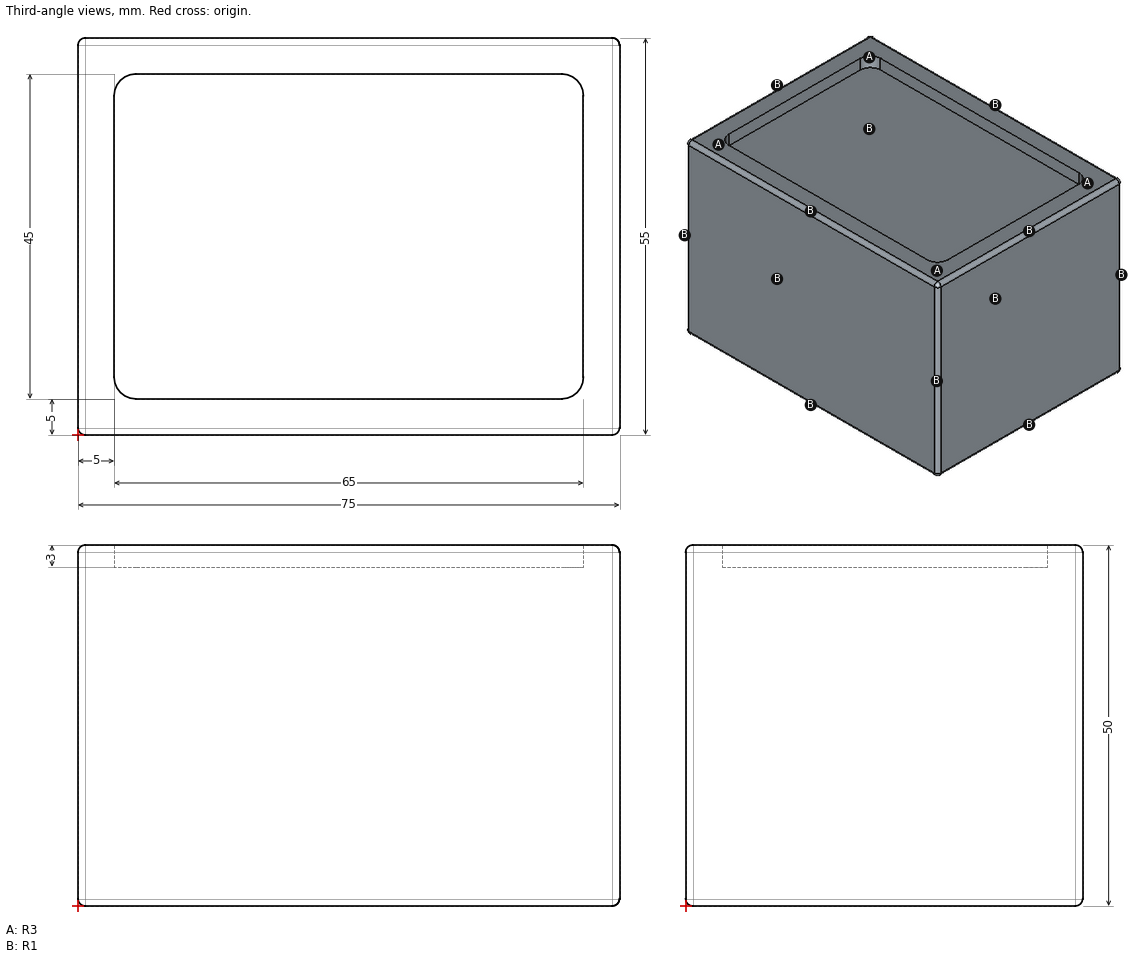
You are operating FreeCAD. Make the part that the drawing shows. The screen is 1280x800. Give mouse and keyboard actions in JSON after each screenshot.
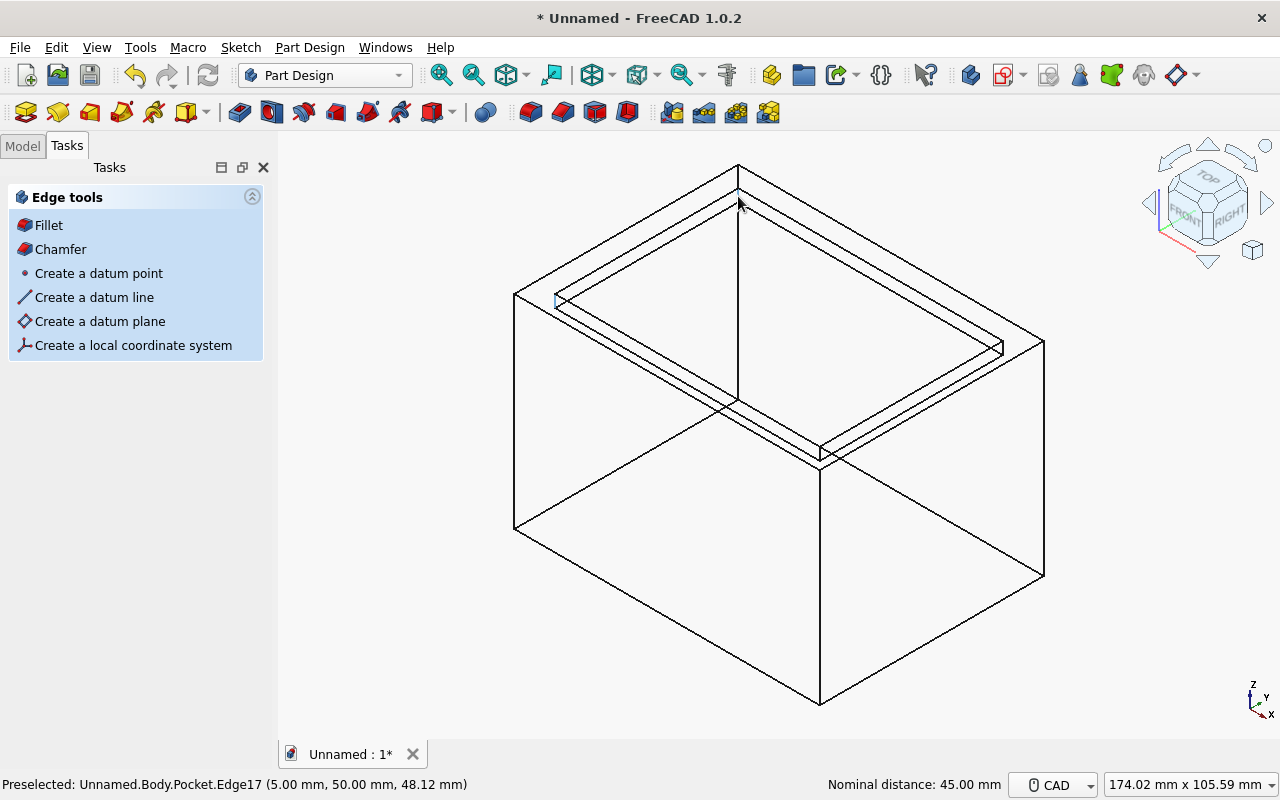
{"action": "left_click", "coordinate": [1003, 348], "text": "ctrl"}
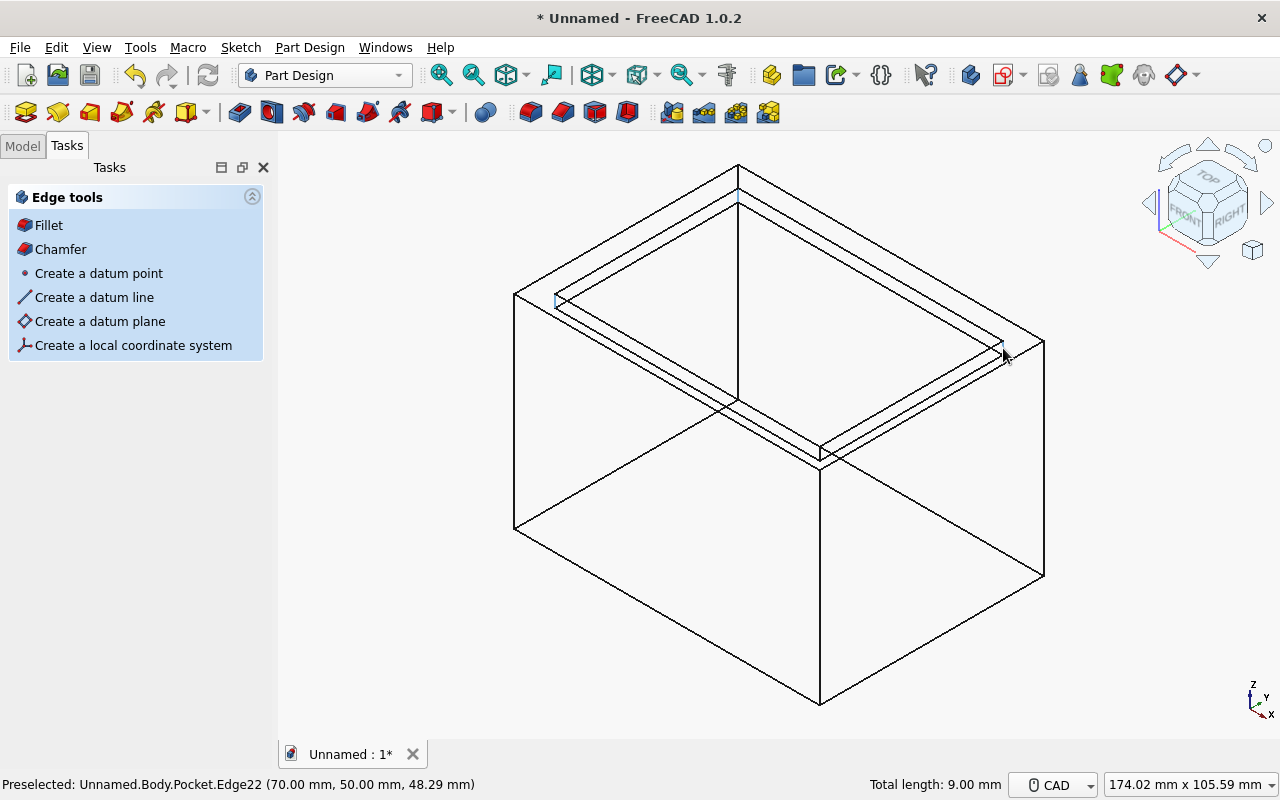
{"action": "left_click", "coordinate": [820, 453], "text": "ctrl"}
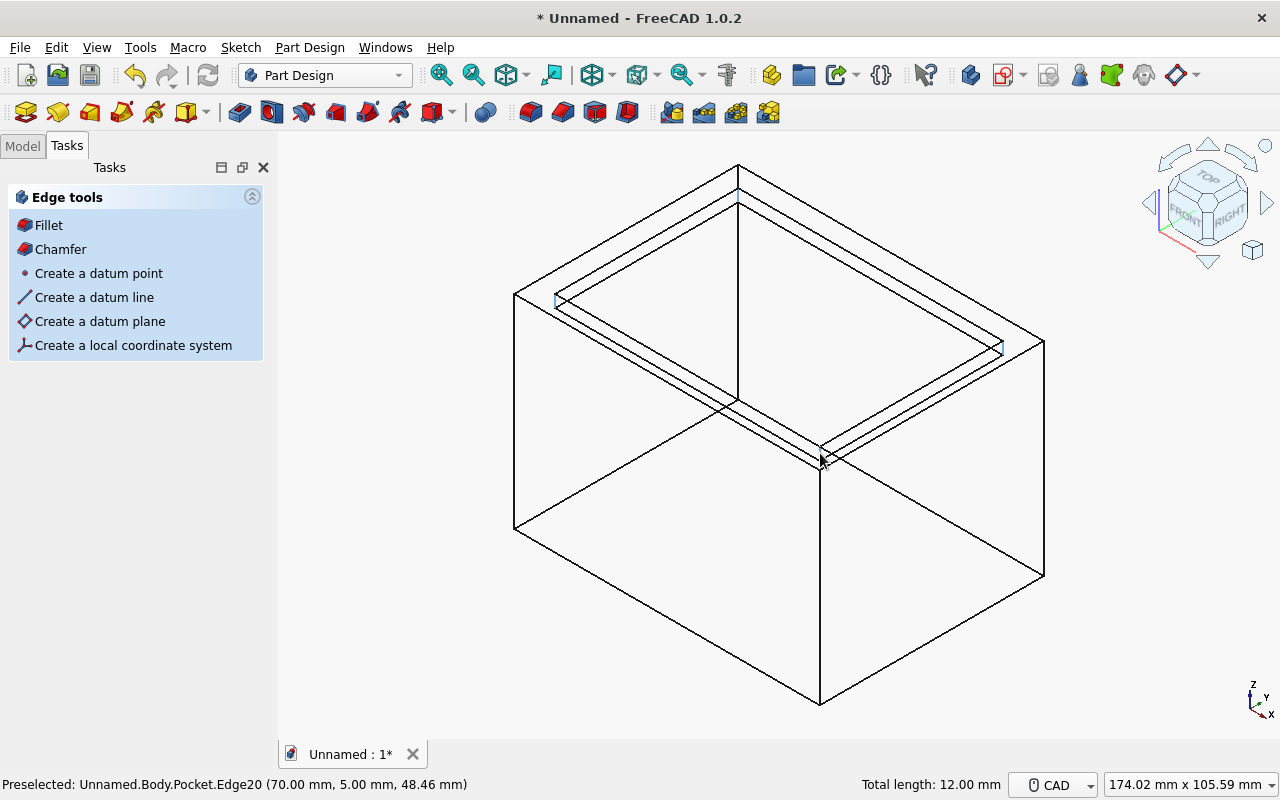
{"action": "key", "text": "v 1"}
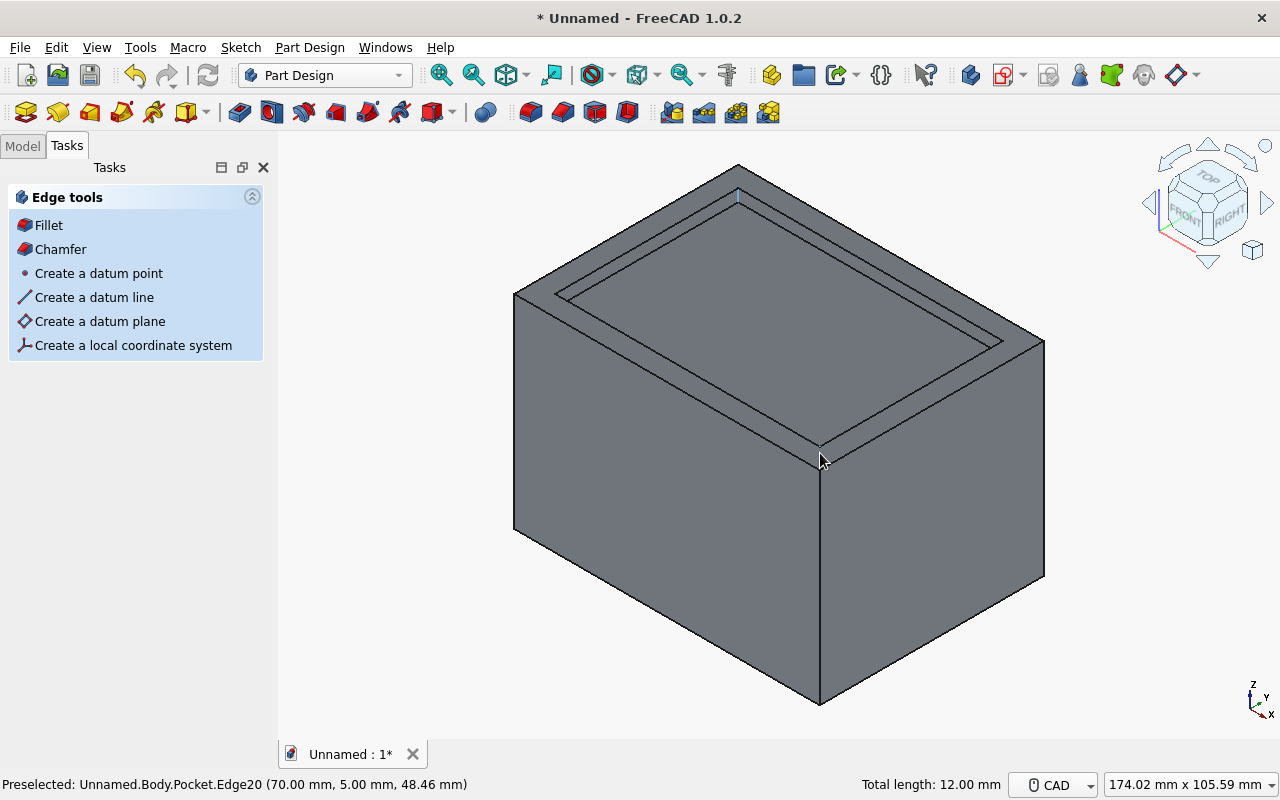
{"action": "left_click", "coordinate": [532, 112]}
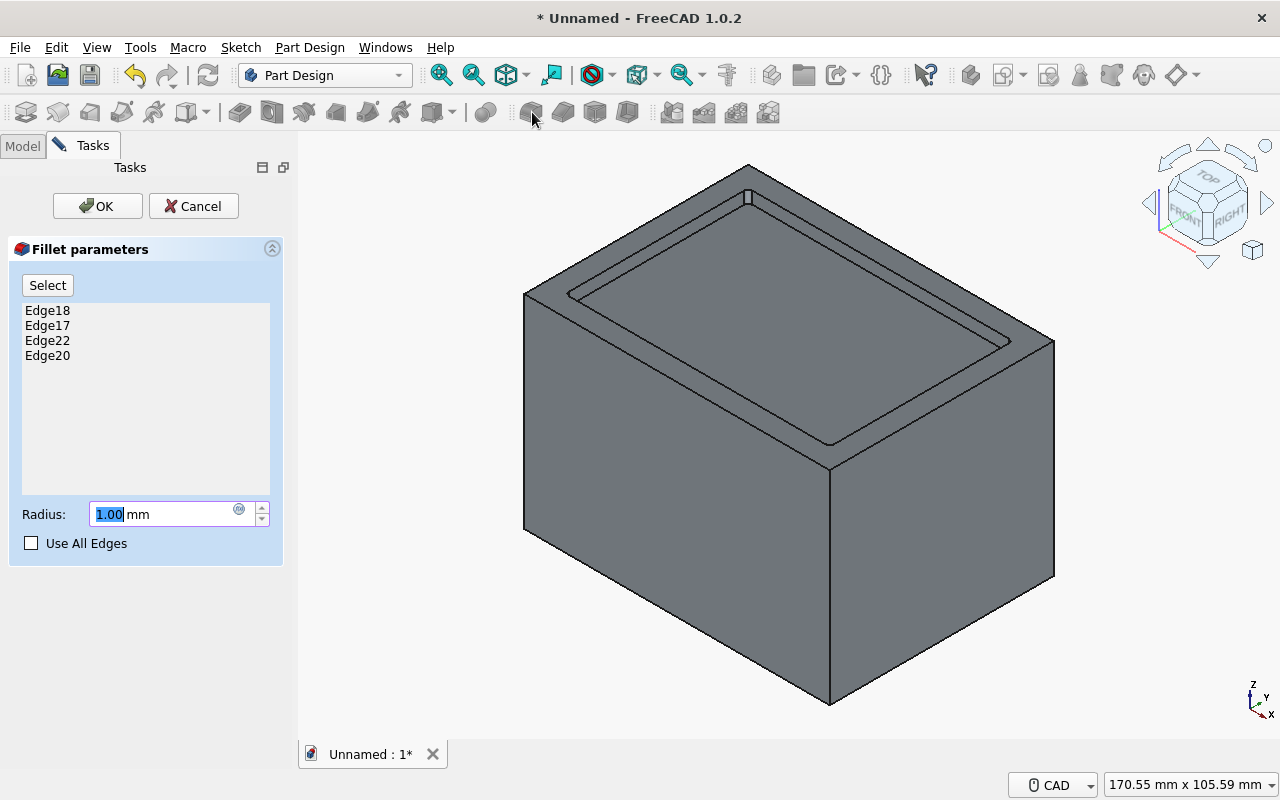
{"action": "type", "text": "3"}
{"action": "key", "text": "Tab"}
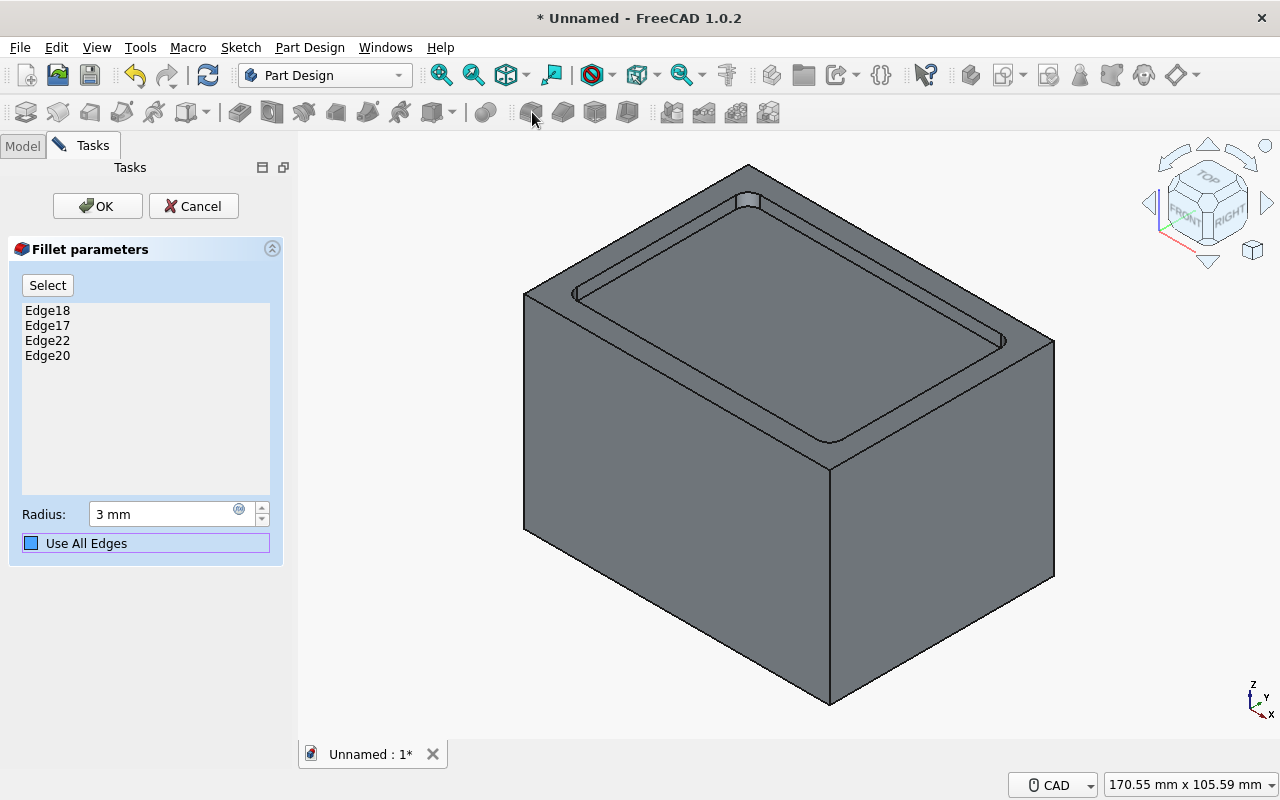
{"action": "left_click", "coordinate": [98, 206]}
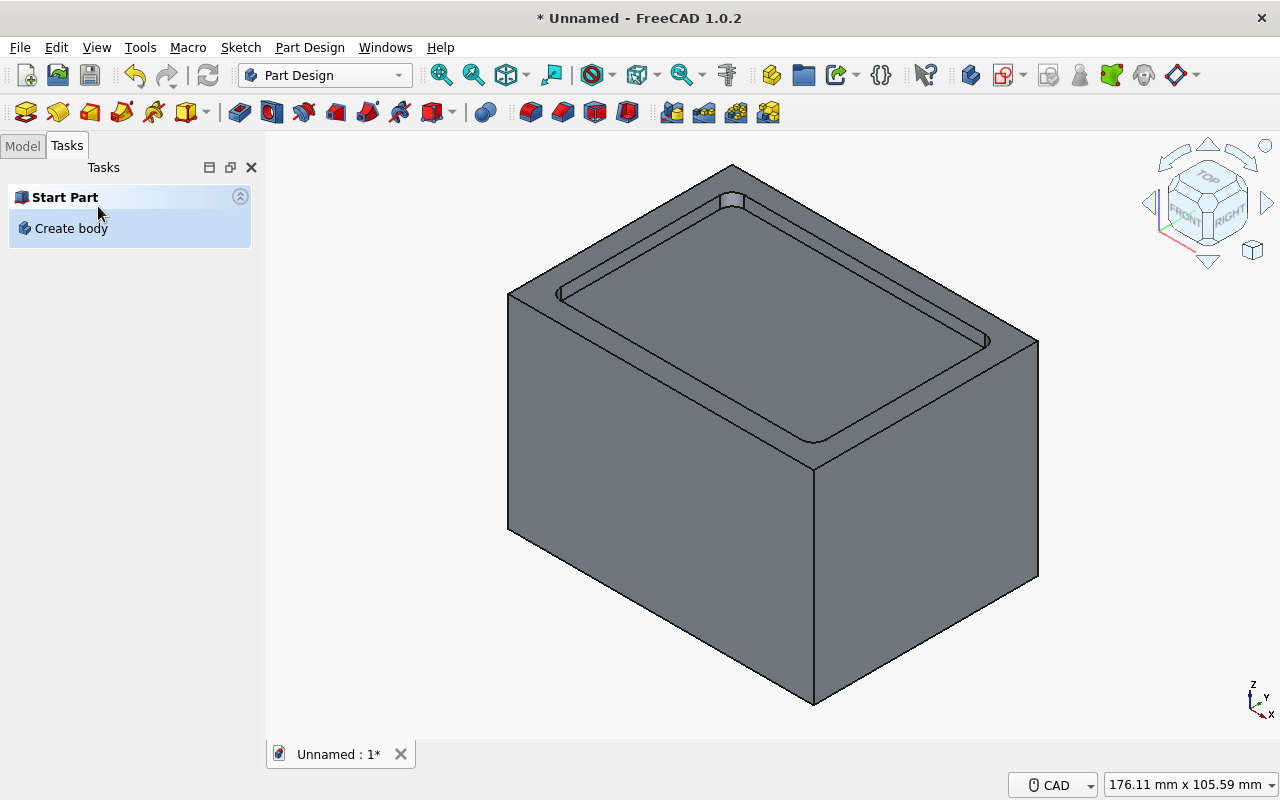
{"action": "left_click", "coordinate": [705, 524]}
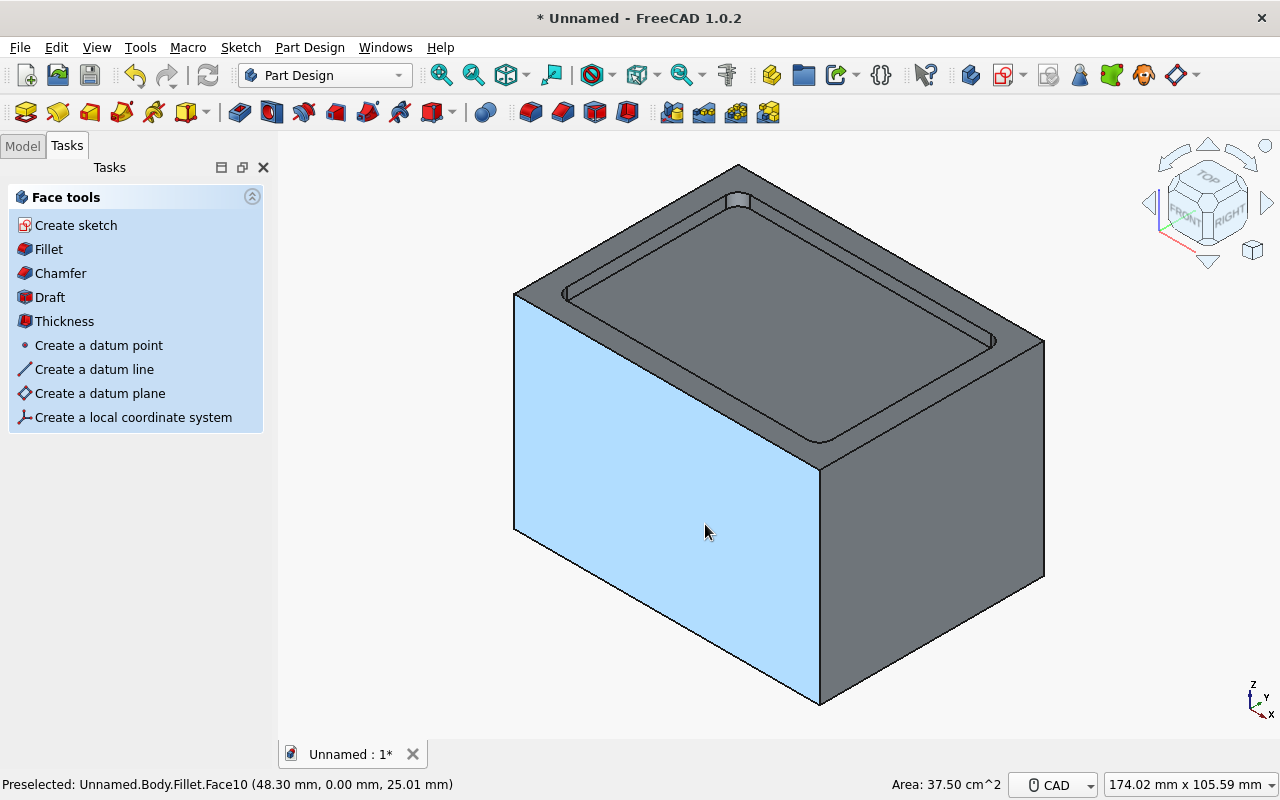
{"action": "left_click", "coordinate": [932, 405], "text": "ctrl"}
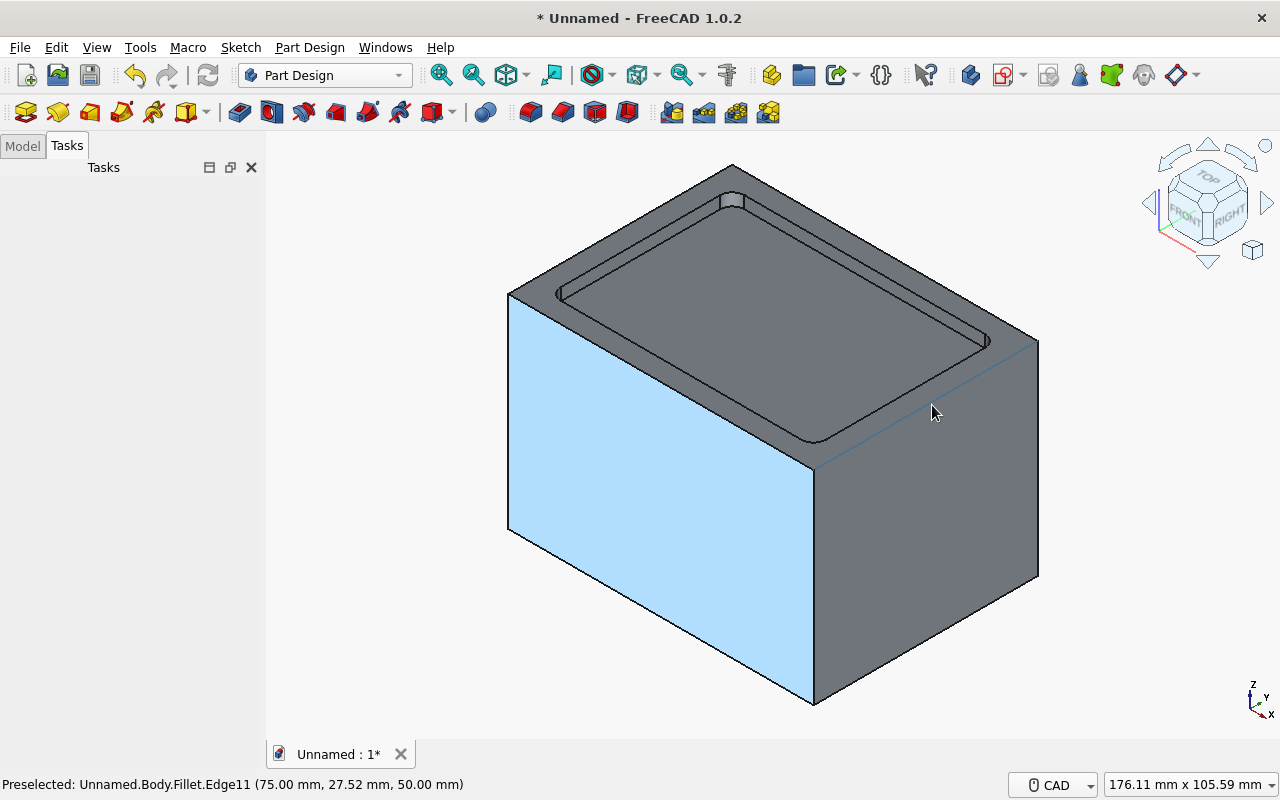
{"action": "key", "text": "2"}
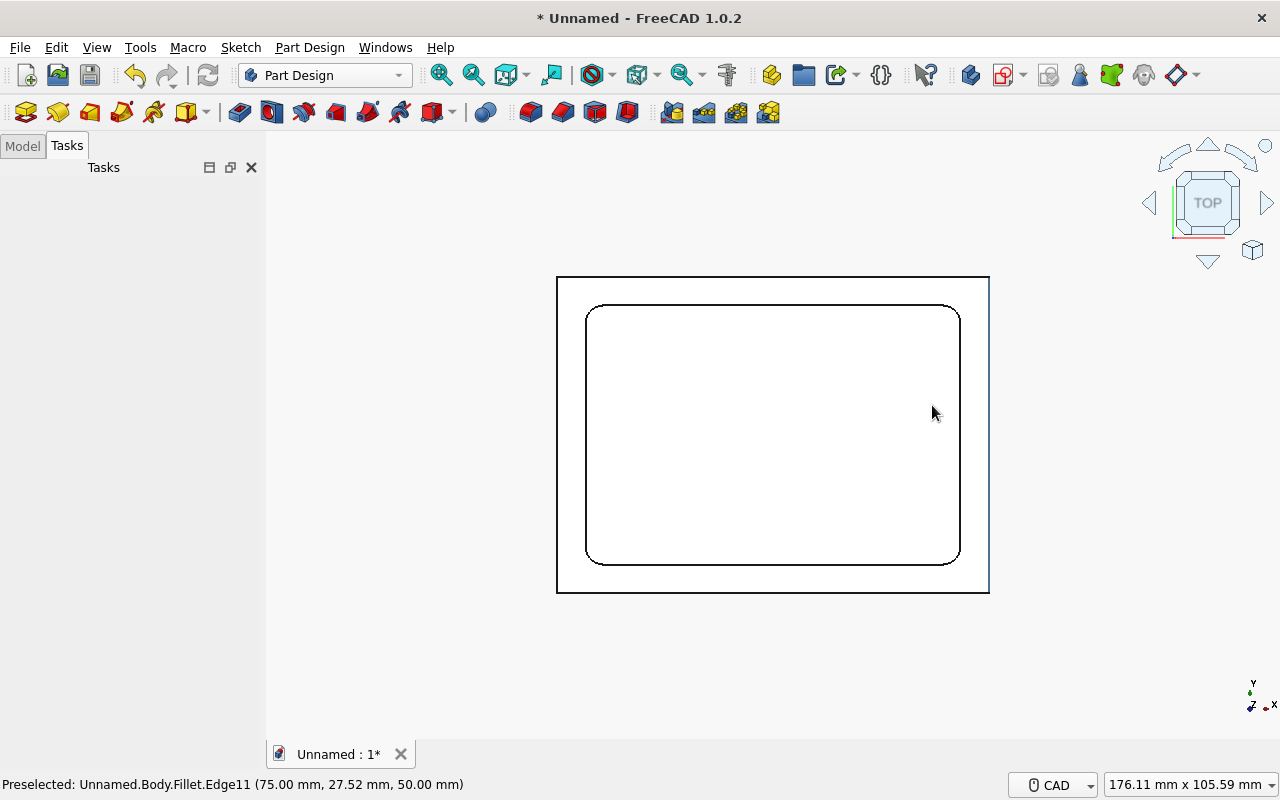
{"action": "left_click", "coordinate": [557, 434], "text": "ctrl"}